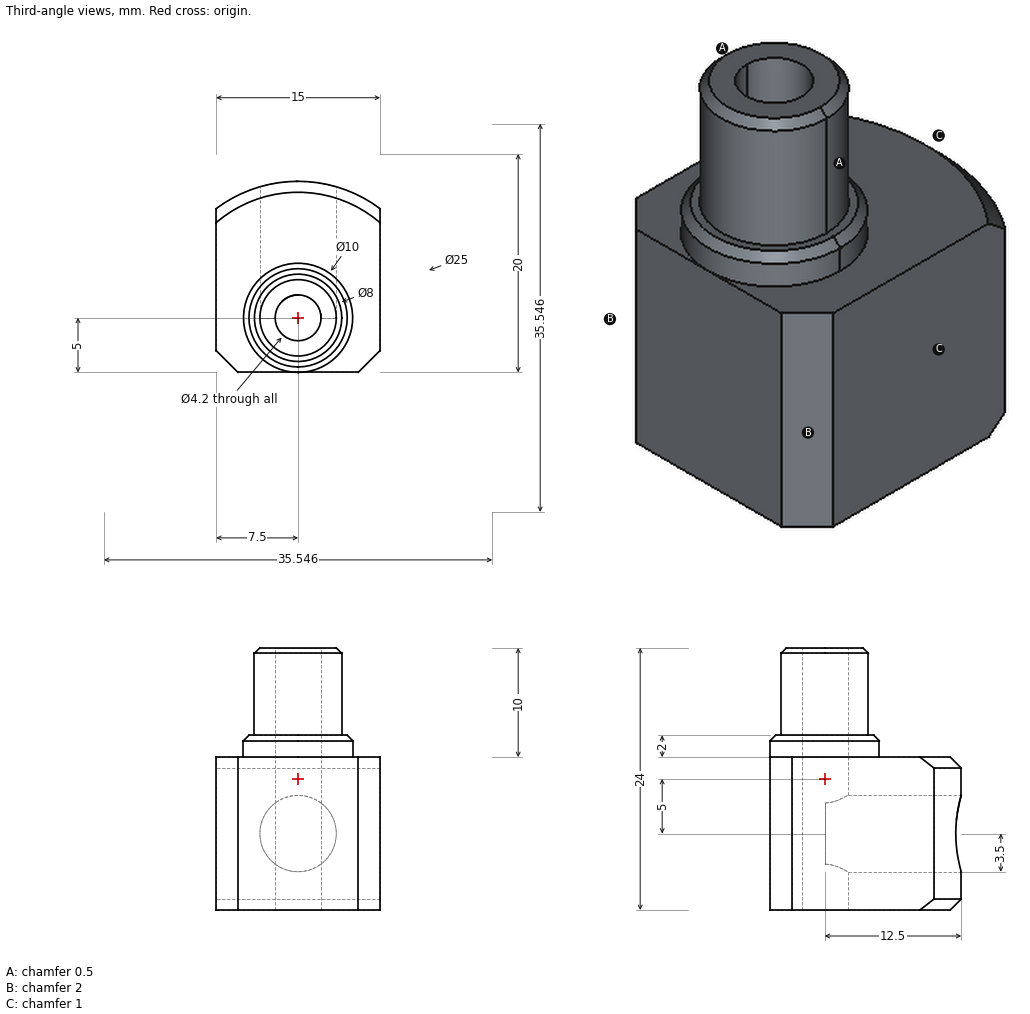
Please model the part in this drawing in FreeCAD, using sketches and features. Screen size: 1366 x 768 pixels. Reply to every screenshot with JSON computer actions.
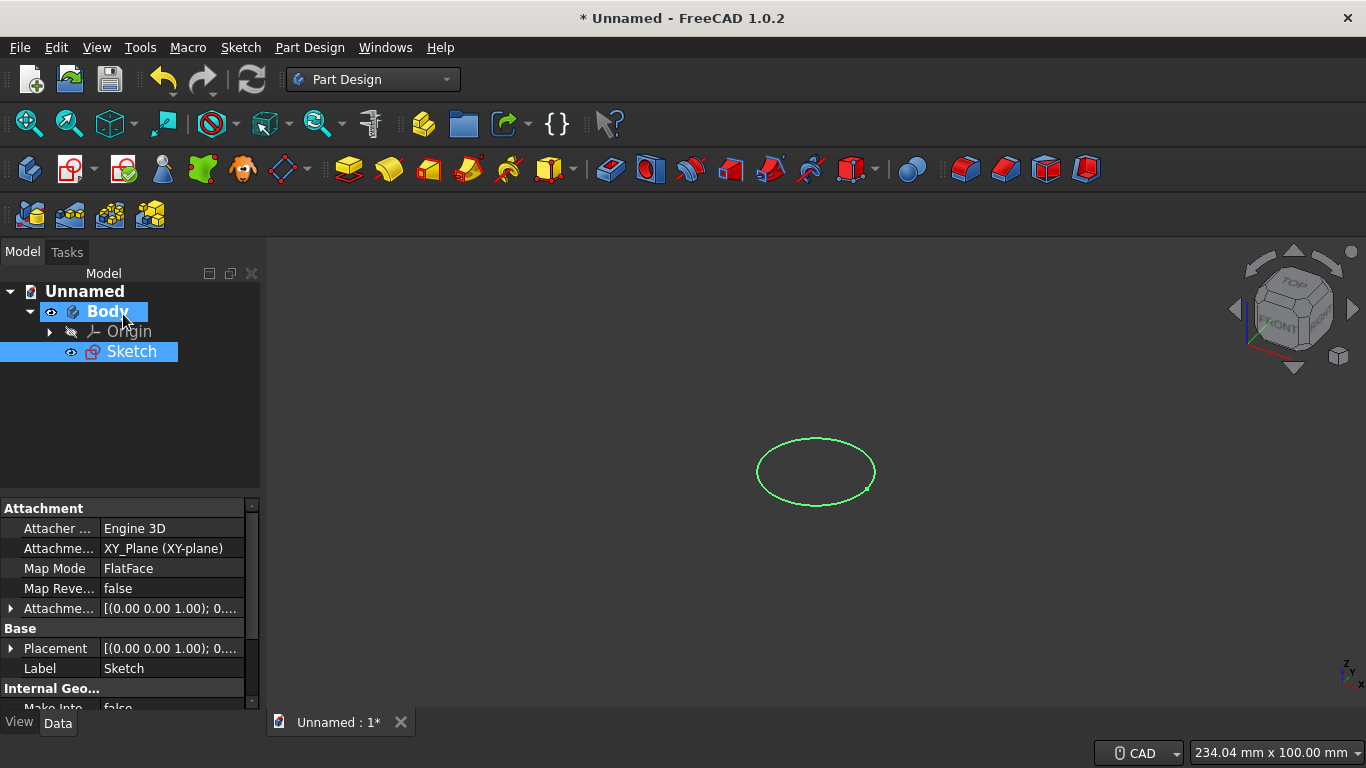
{"action": "left_click", "coordinate": [350, 170]}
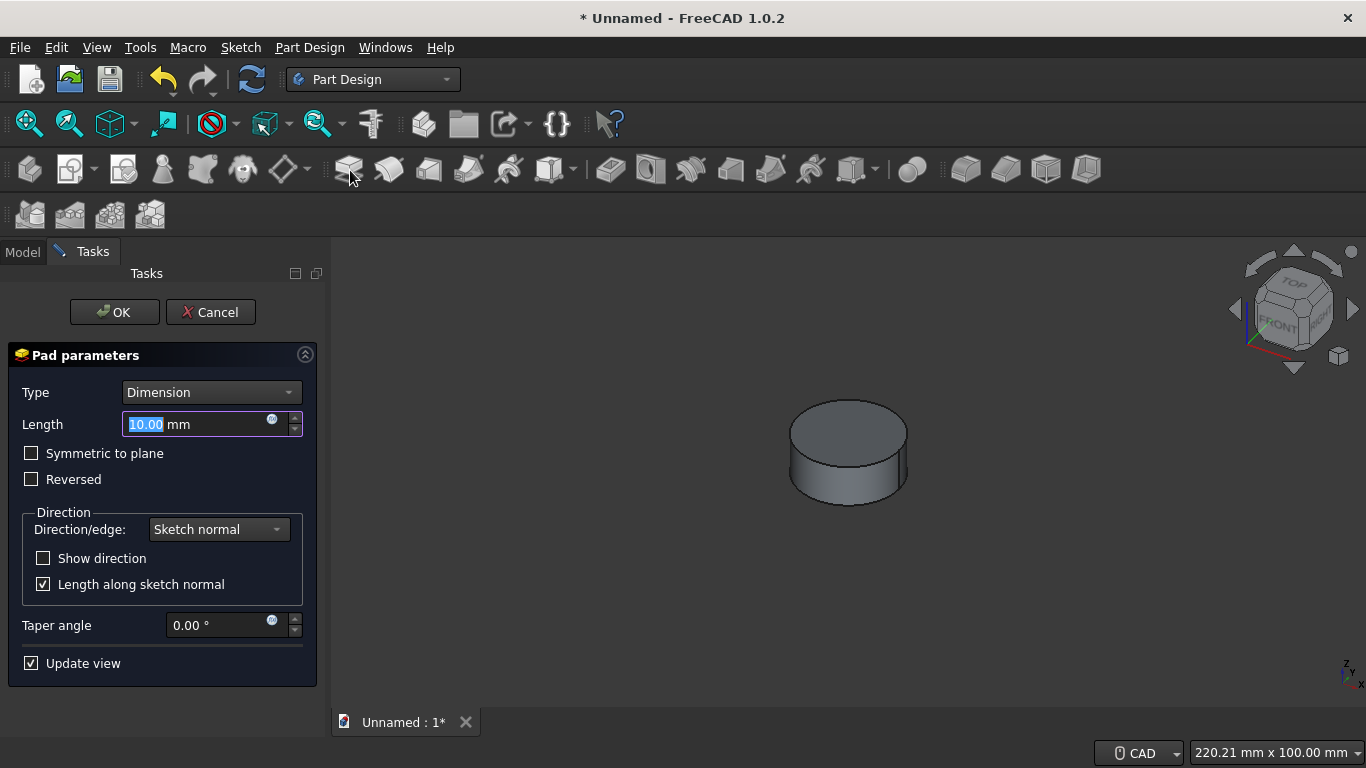
{"action": "type", "text": "24"}
{"action": "key", "text": "Tab"}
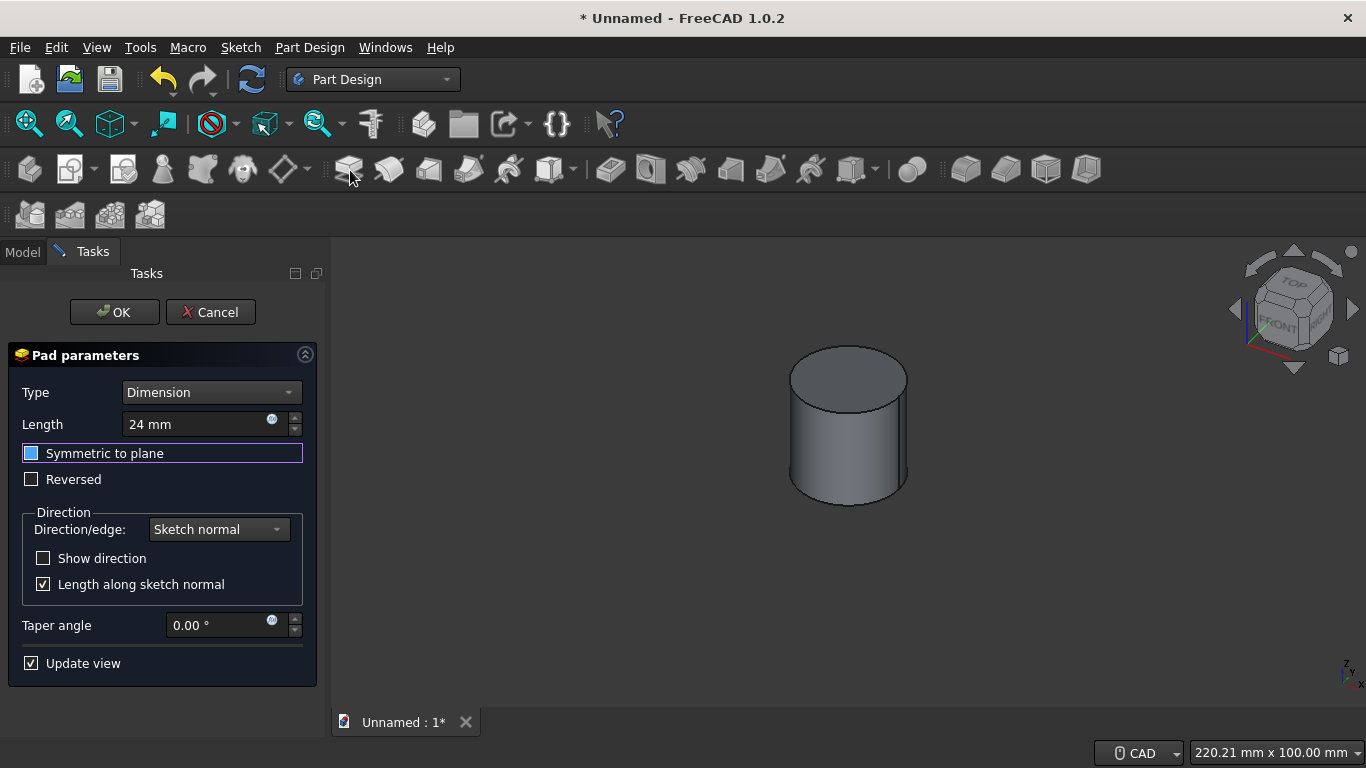
{"action": "left_click", "coordinate": [30, 453]}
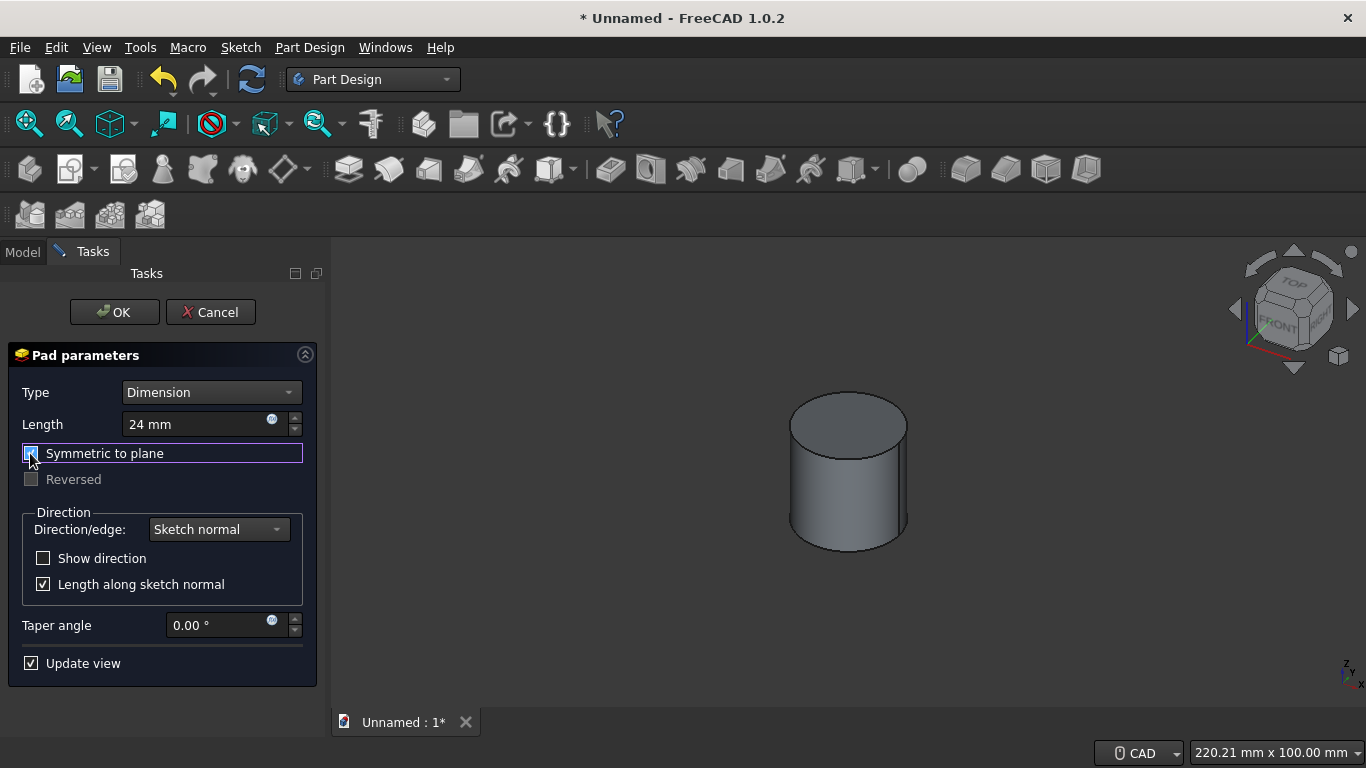
{"action": "left_click", "coordinate": [115, 312]}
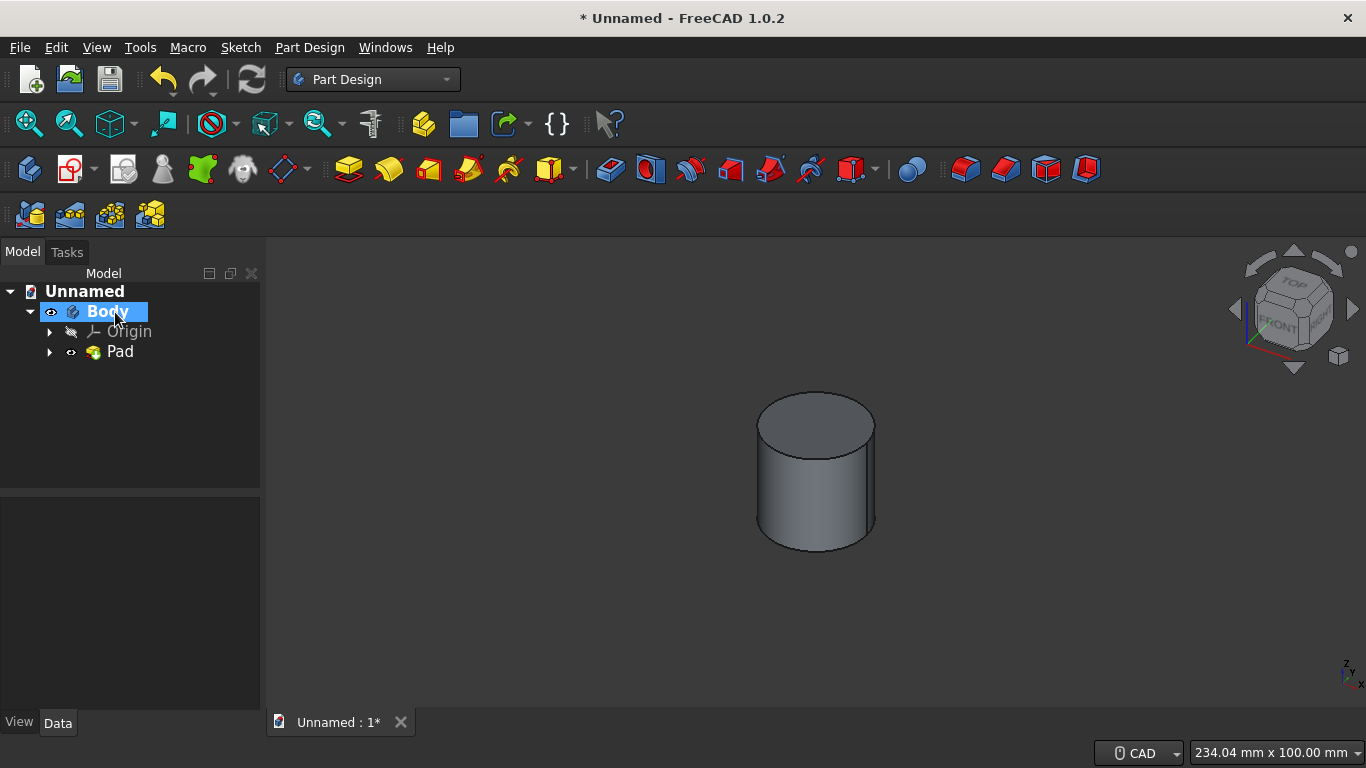
{"action": "left_click", "coordinate": [30, 124]}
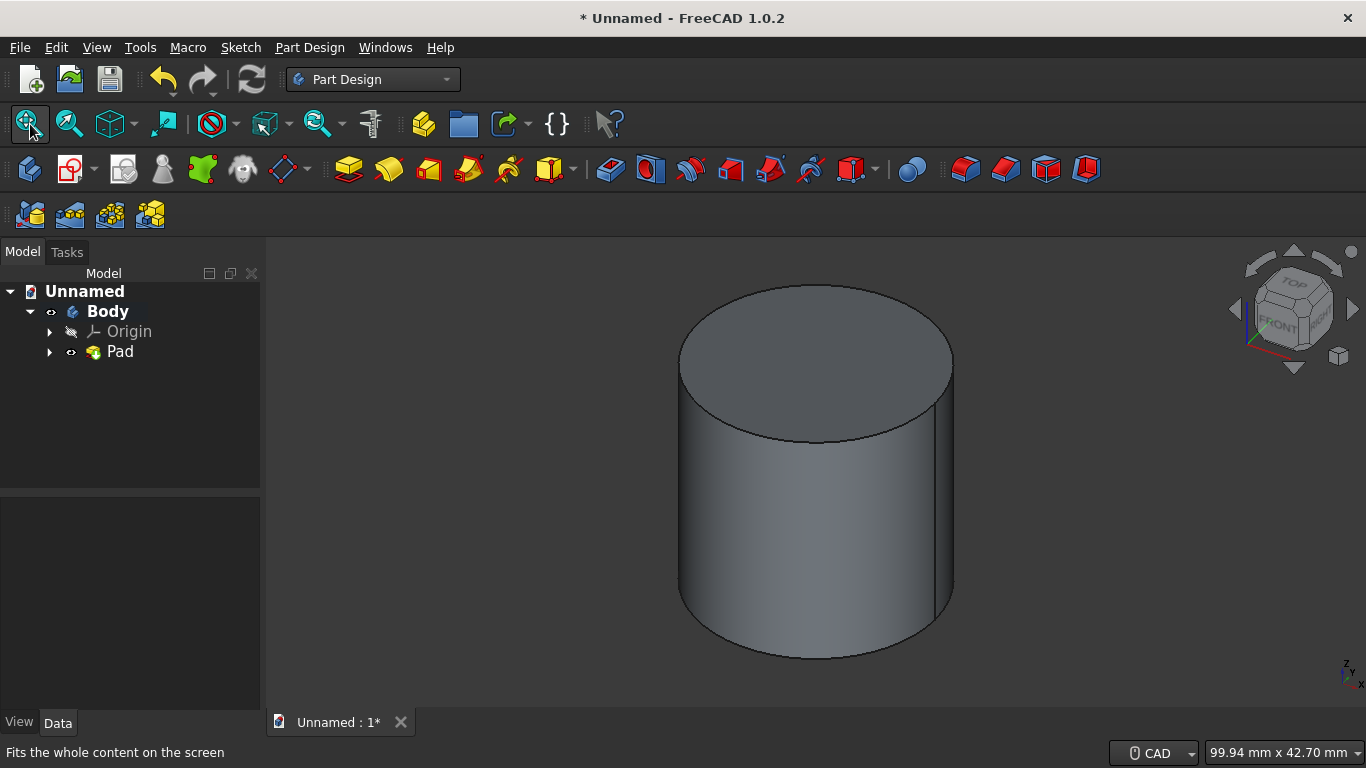
{"action": "left_click", "coordinate": [816, 363]}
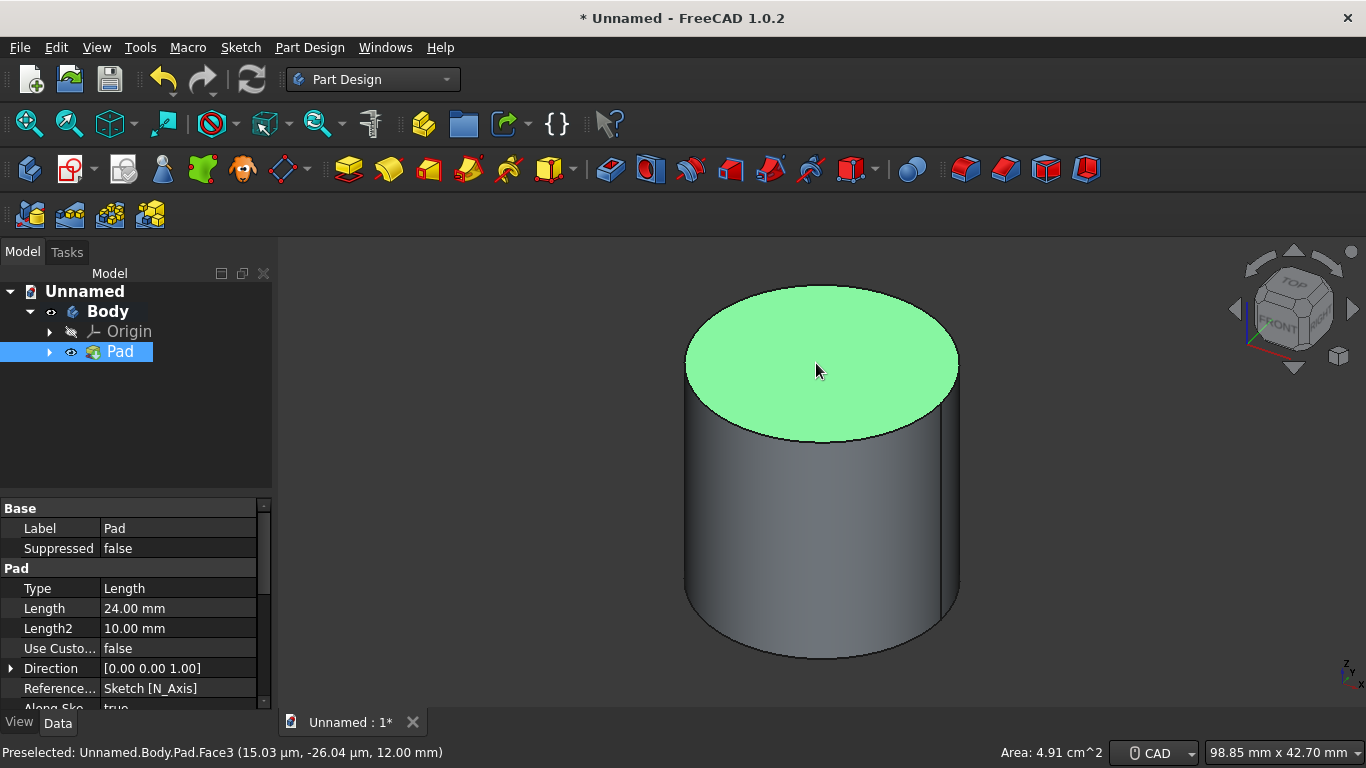
{"action": "left_click", "coordinate": [70, 170]}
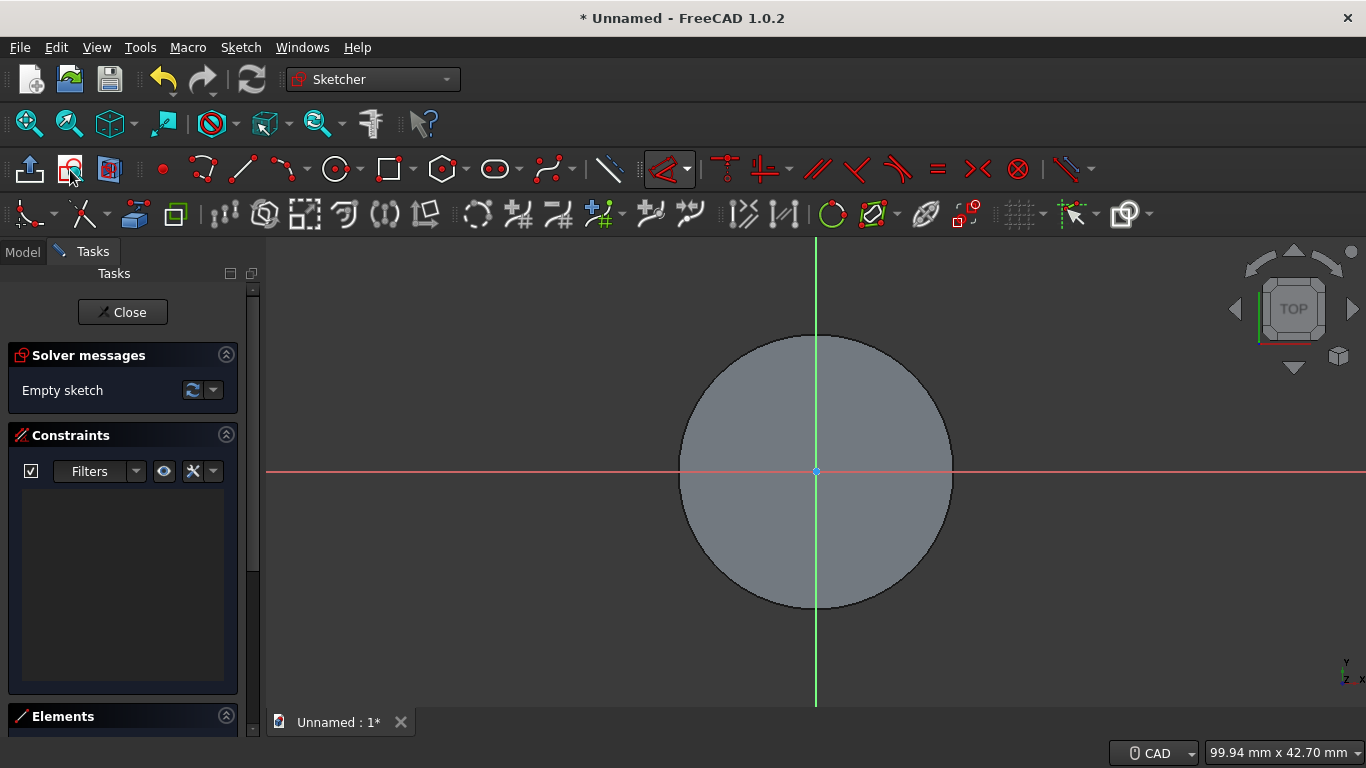
{"action": "scroll", "coordinate": [438, 472], "scroll_direction": "down", "scroll_amount": 1}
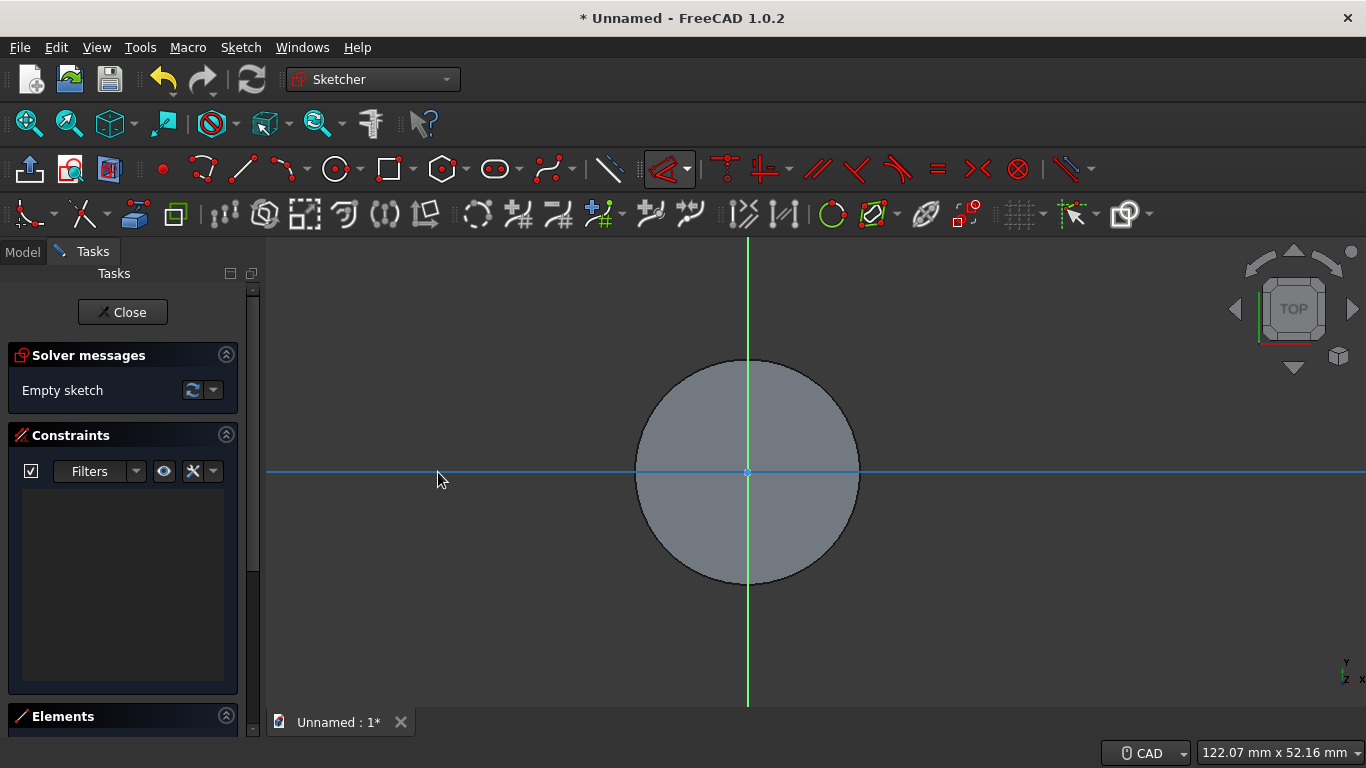
{"action": "key", "text": "g v"}